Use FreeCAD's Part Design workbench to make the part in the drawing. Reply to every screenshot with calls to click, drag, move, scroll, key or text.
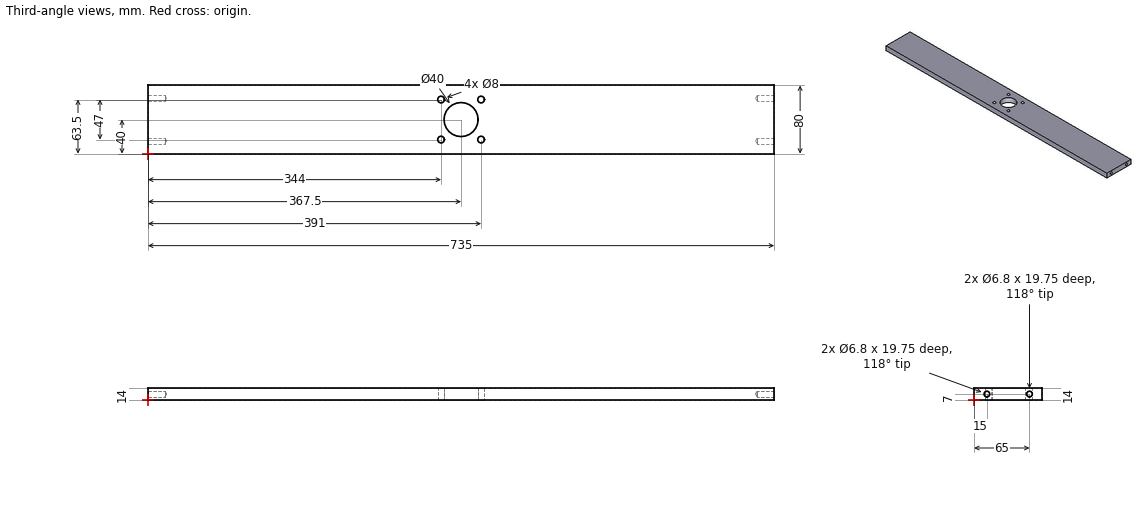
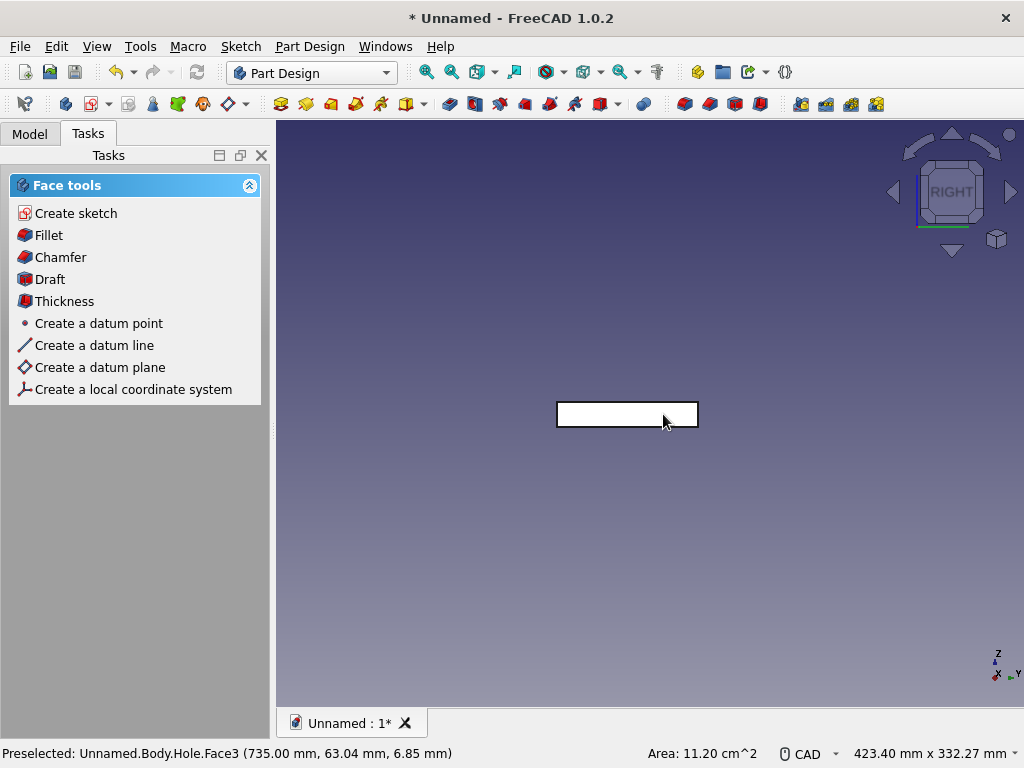
click(90, 104)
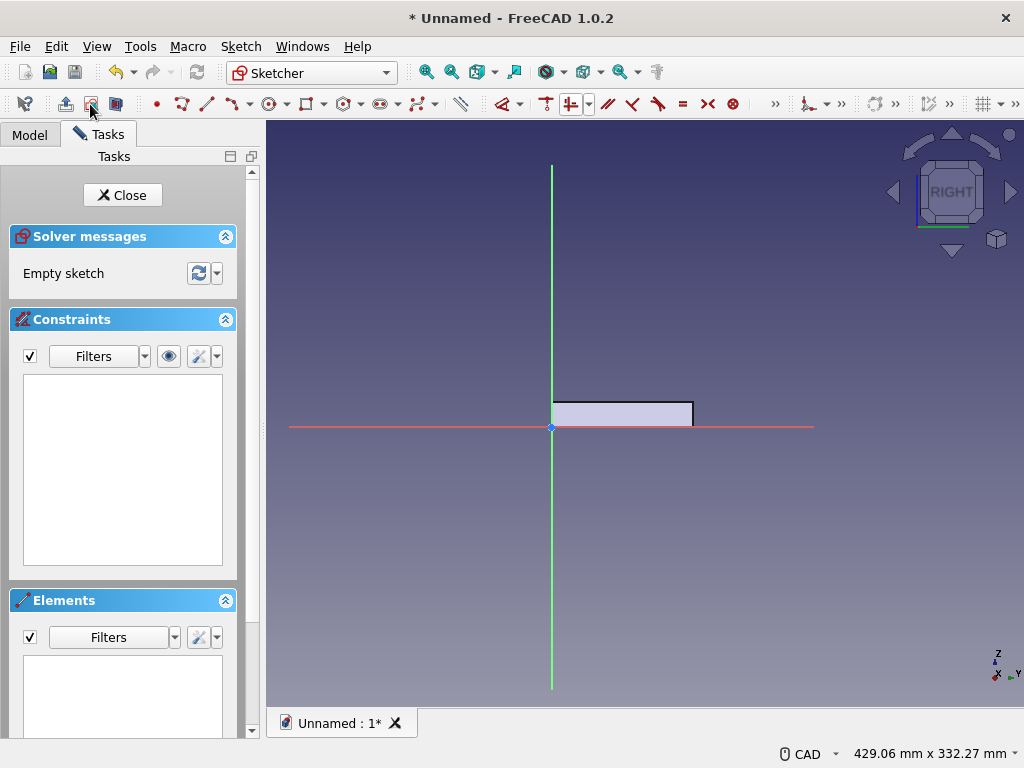
scroll(627, 420, up, 6)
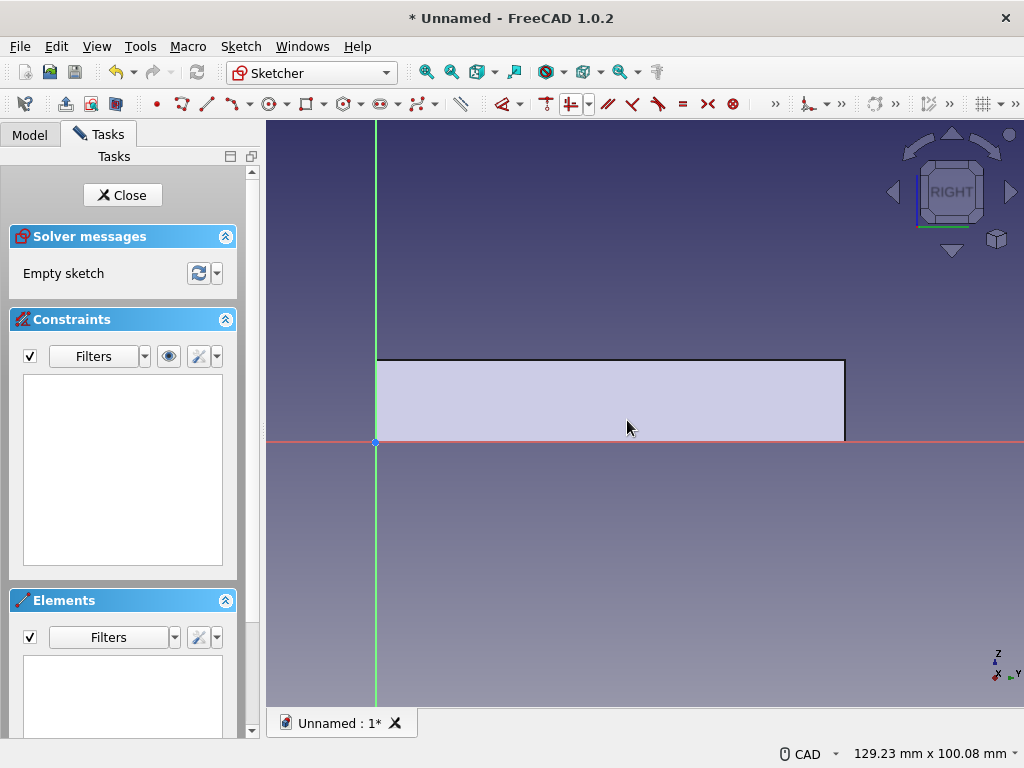
key(g)
key(c)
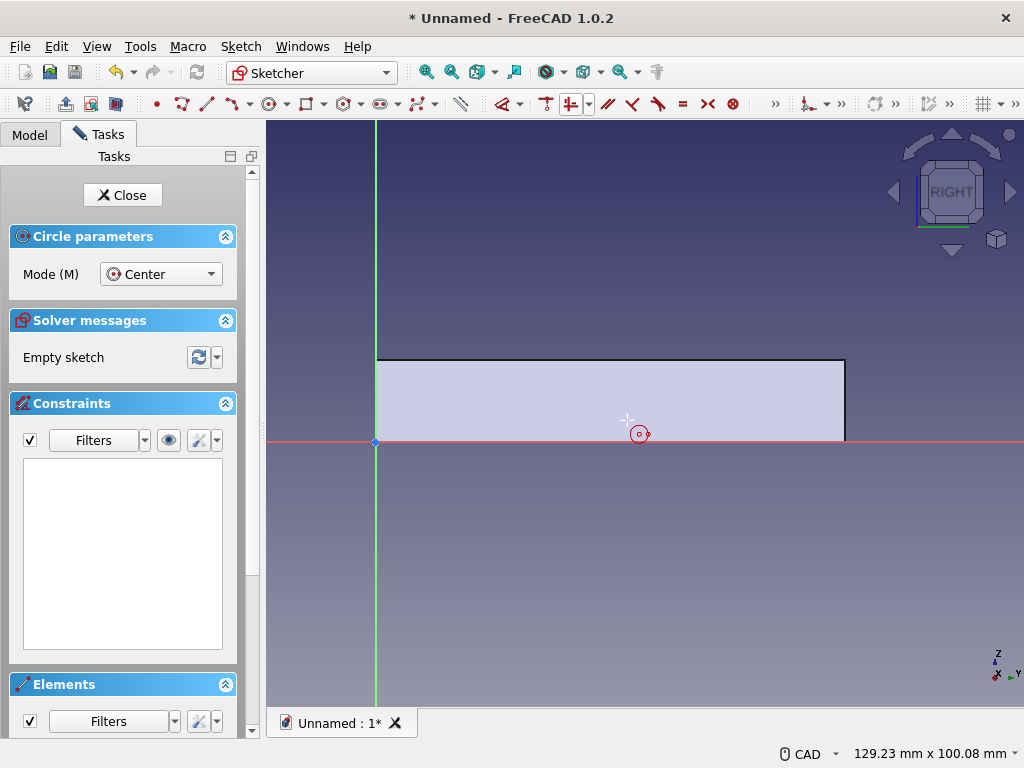
click(464, 401)
move(478, 387)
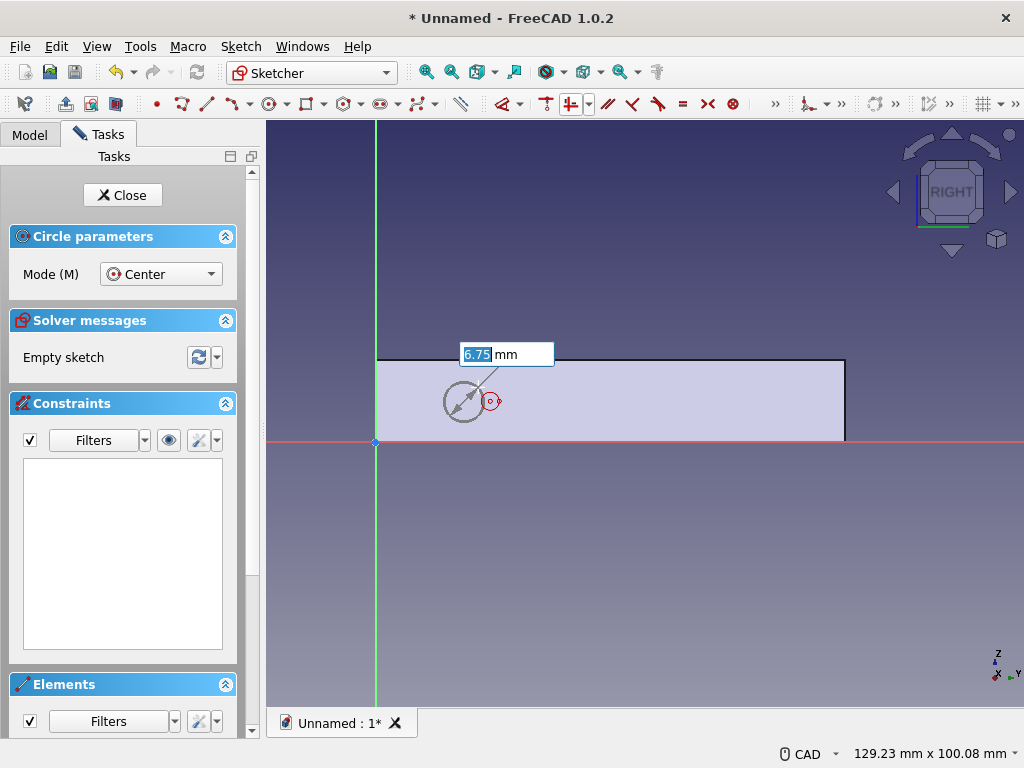
text(6.8)
key(Return)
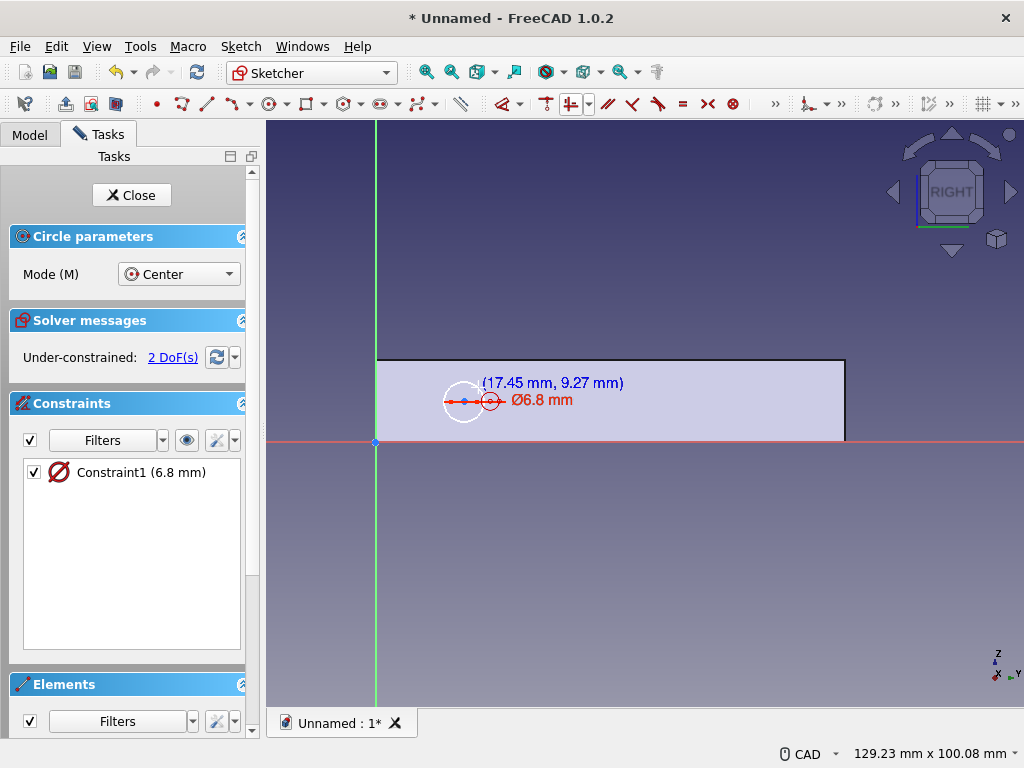
click(757, 401)
move(771, 387)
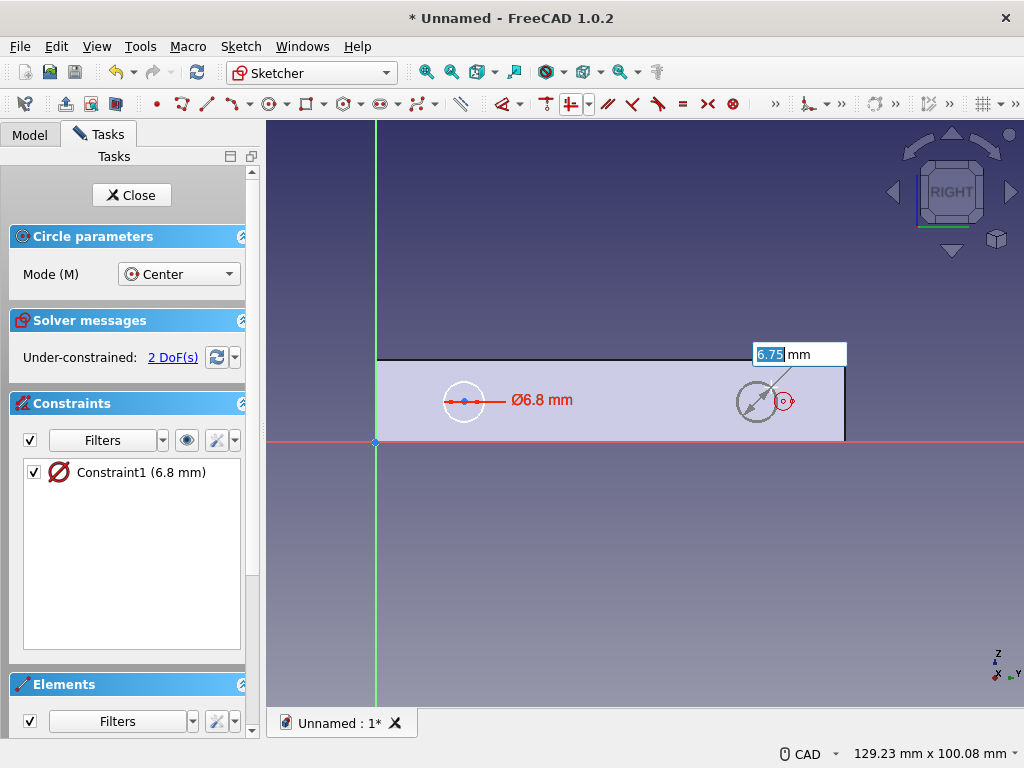
text(6.8)
key(Return)
key(Escape)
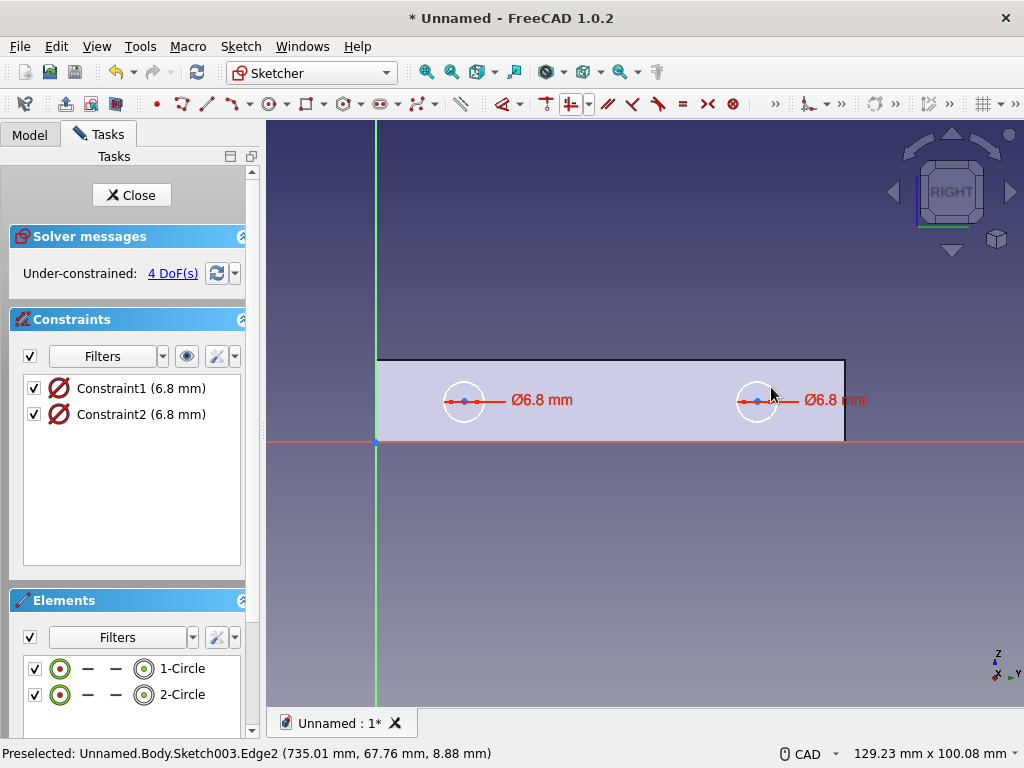
click(464, 402)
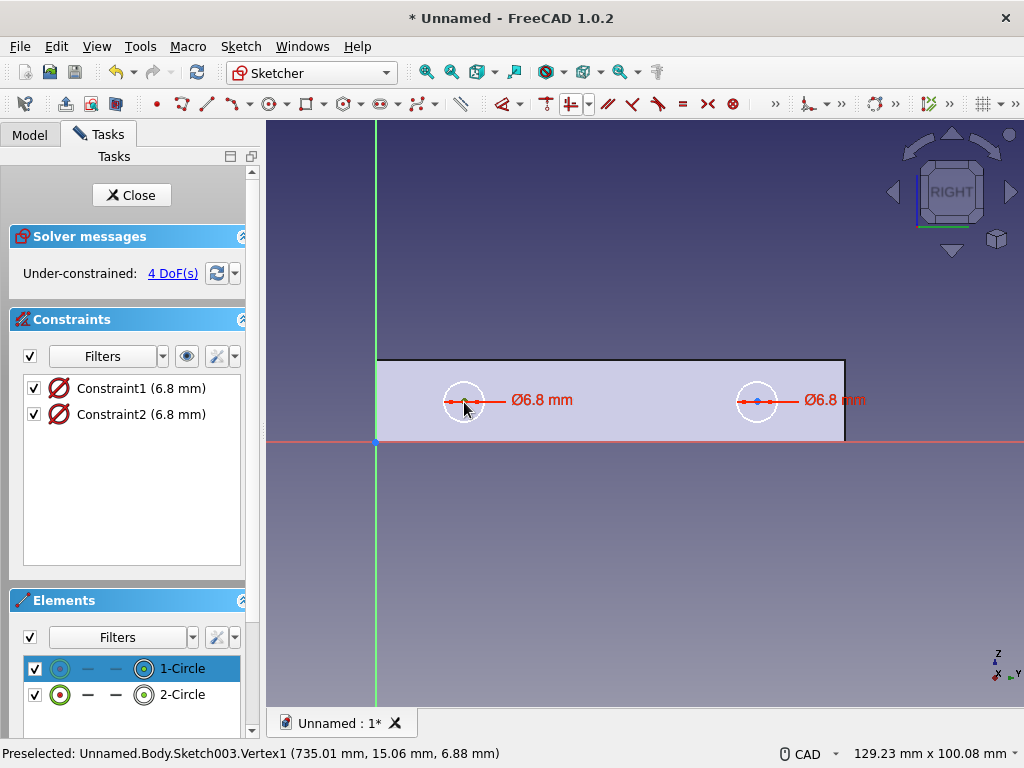
click(757, 402)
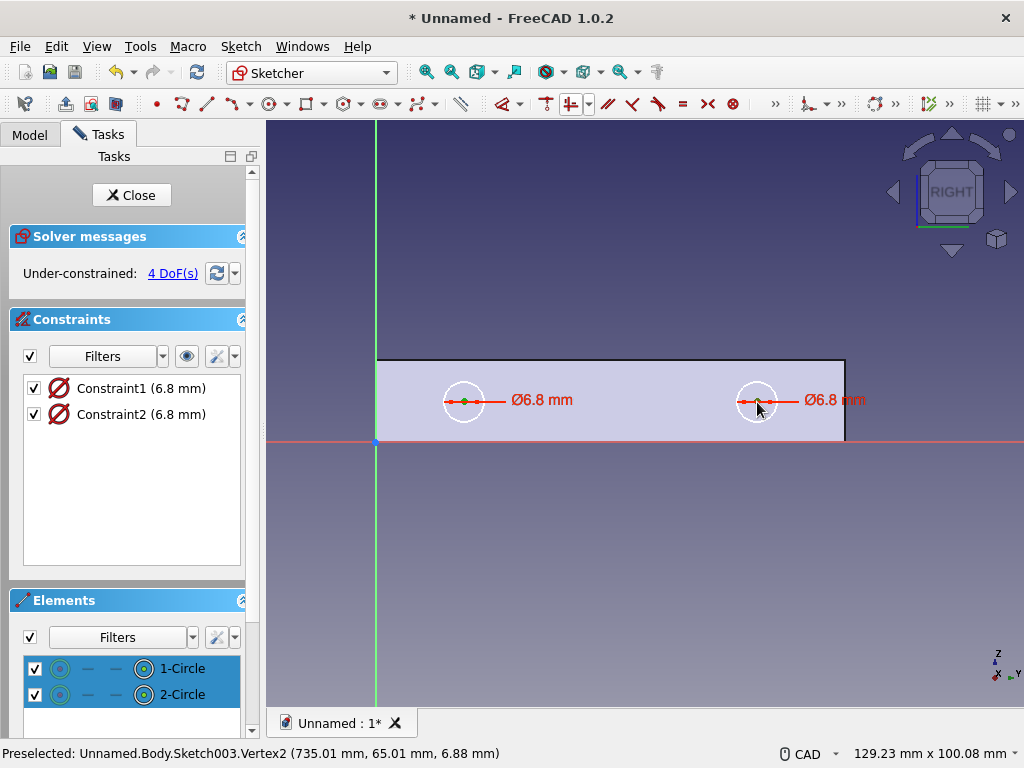
key(h)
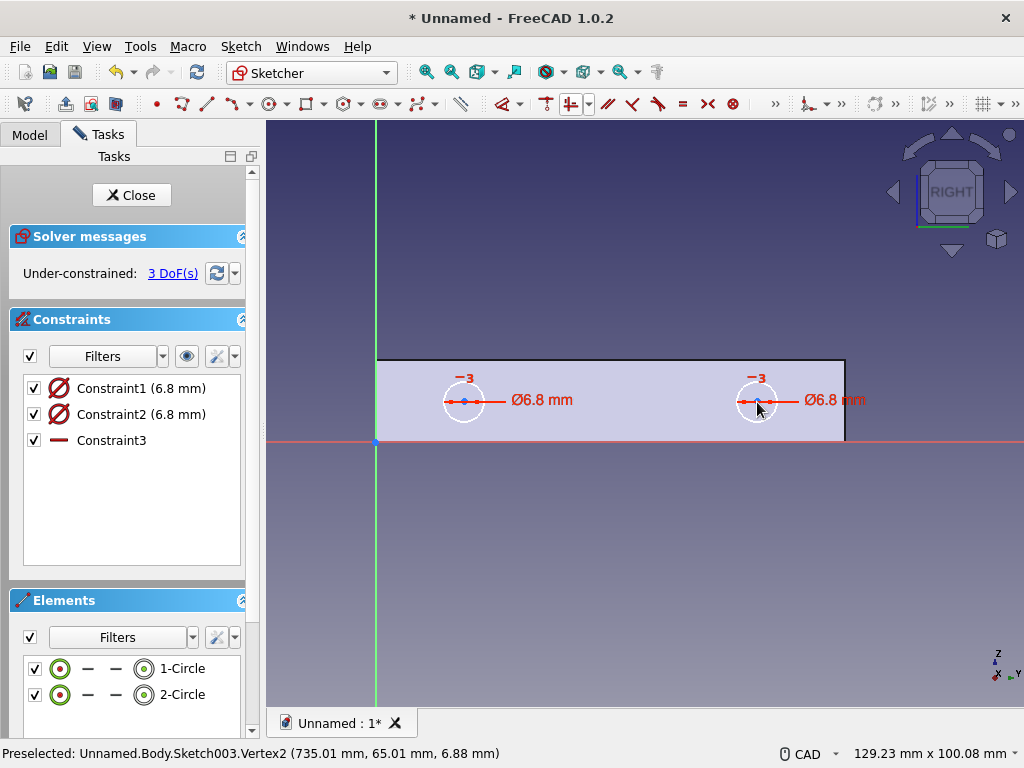
key(d)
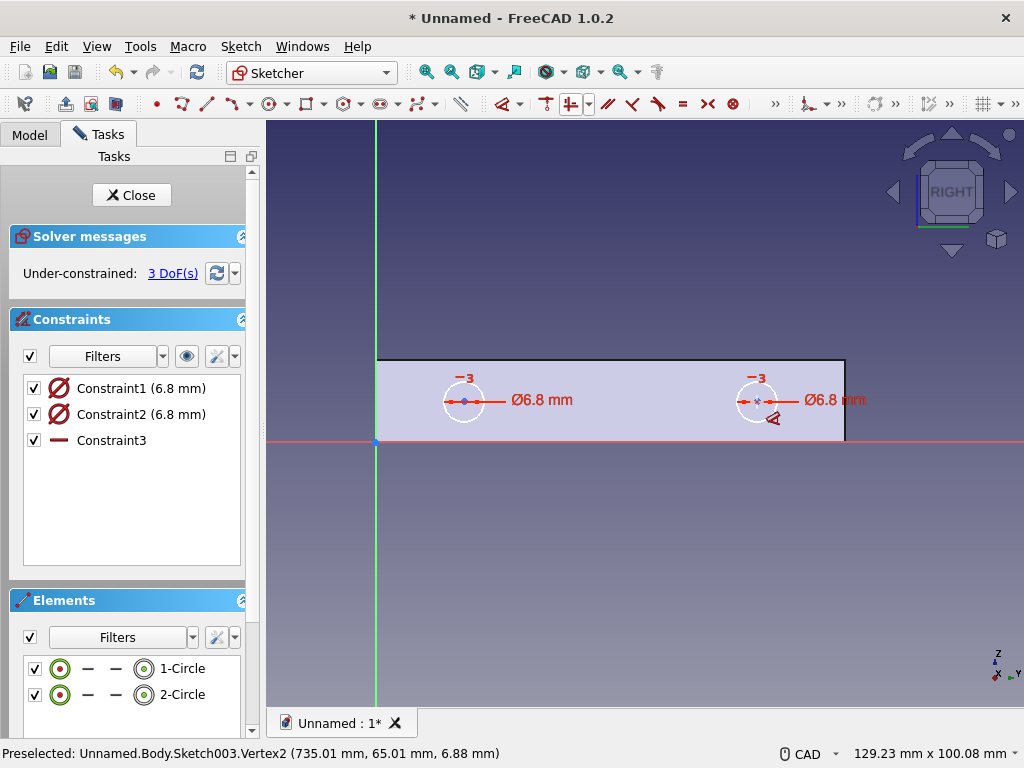
click(464, 402)
click(342, 422)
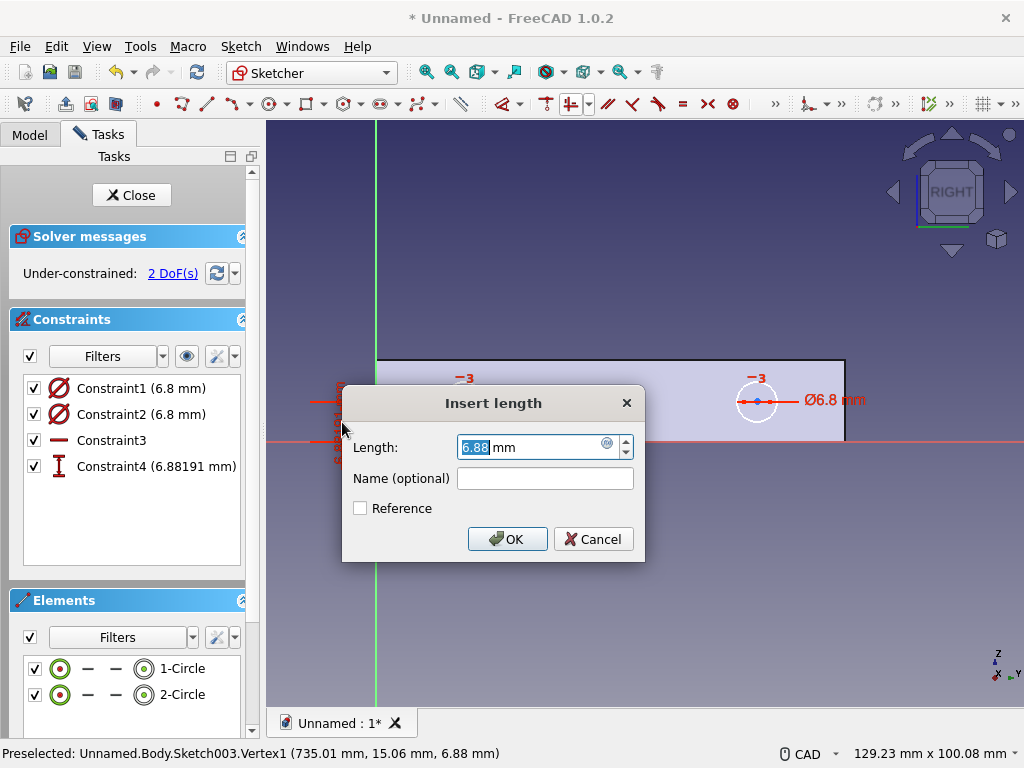
text(7)
key(Return)